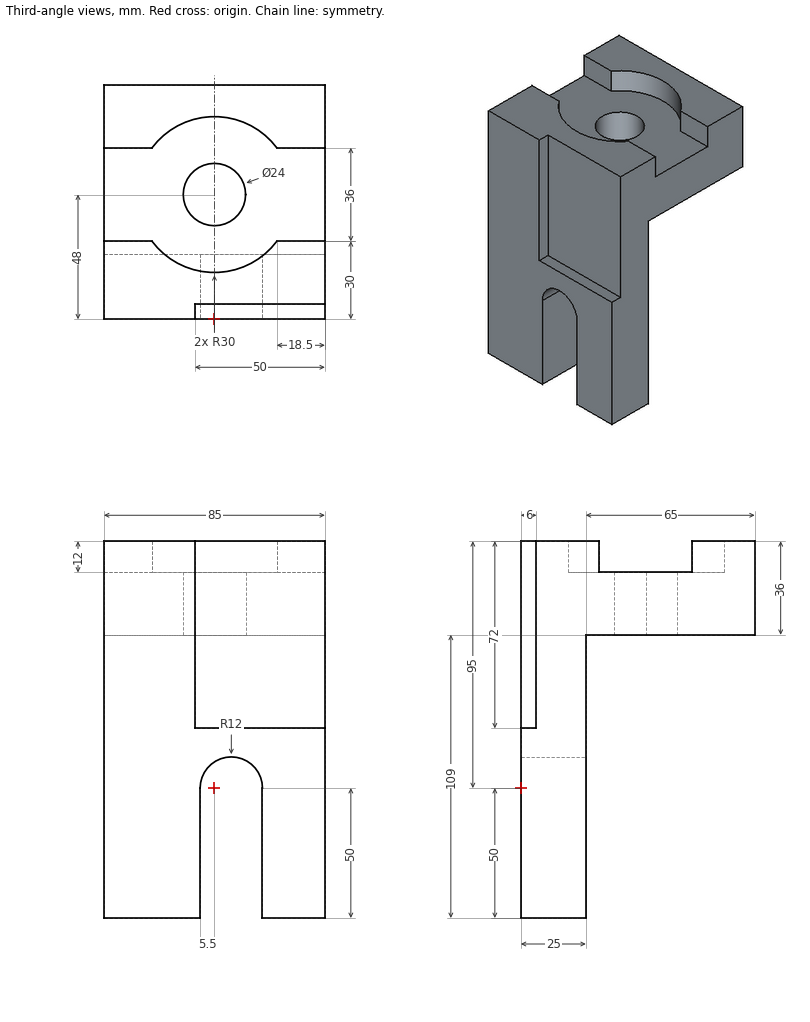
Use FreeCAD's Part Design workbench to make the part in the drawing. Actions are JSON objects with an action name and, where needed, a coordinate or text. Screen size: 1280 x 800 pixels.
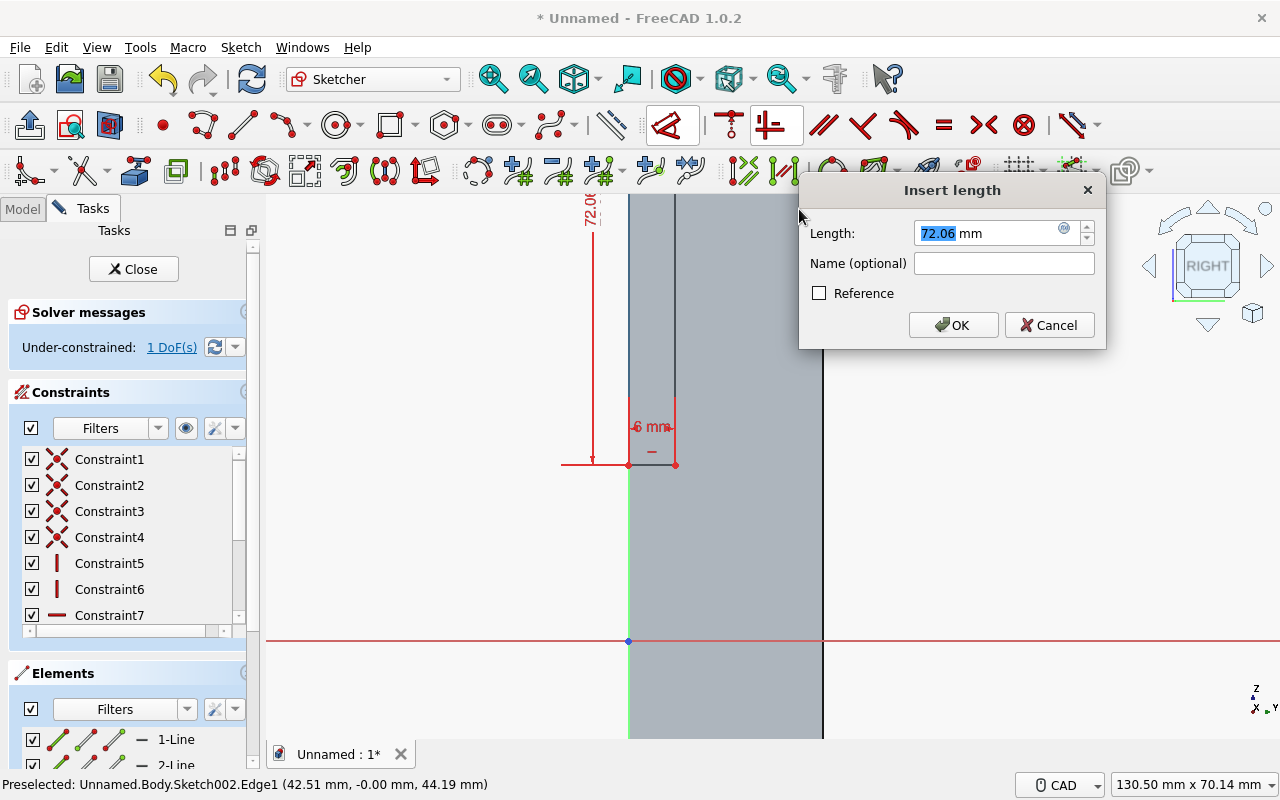
{"action": "type", "text": "72"}
{"action": "key", "text": "Return"}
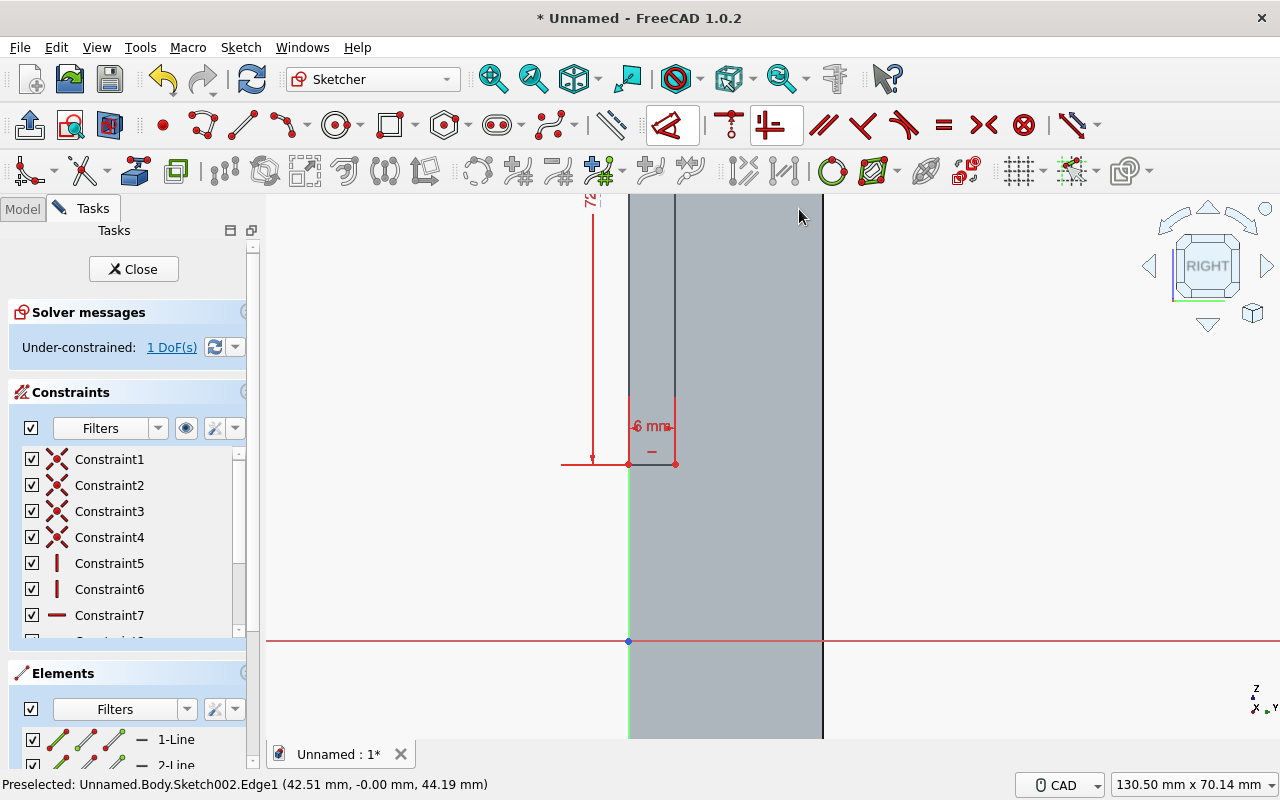
{"action": "scroll", "coordinate": [747, 625], "scroll_direction": "down", "scroll_amount": 4}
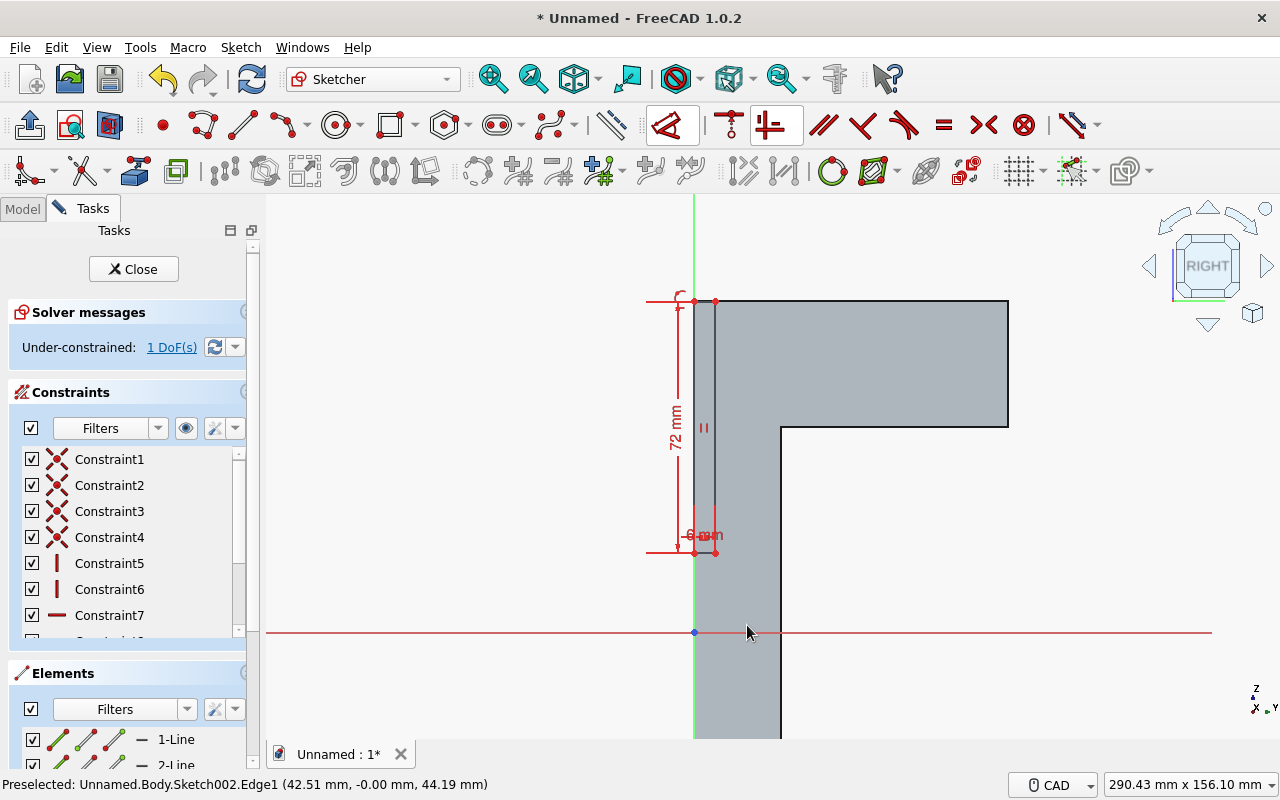
{"action": "left_click", "coordinate": [694, 302]}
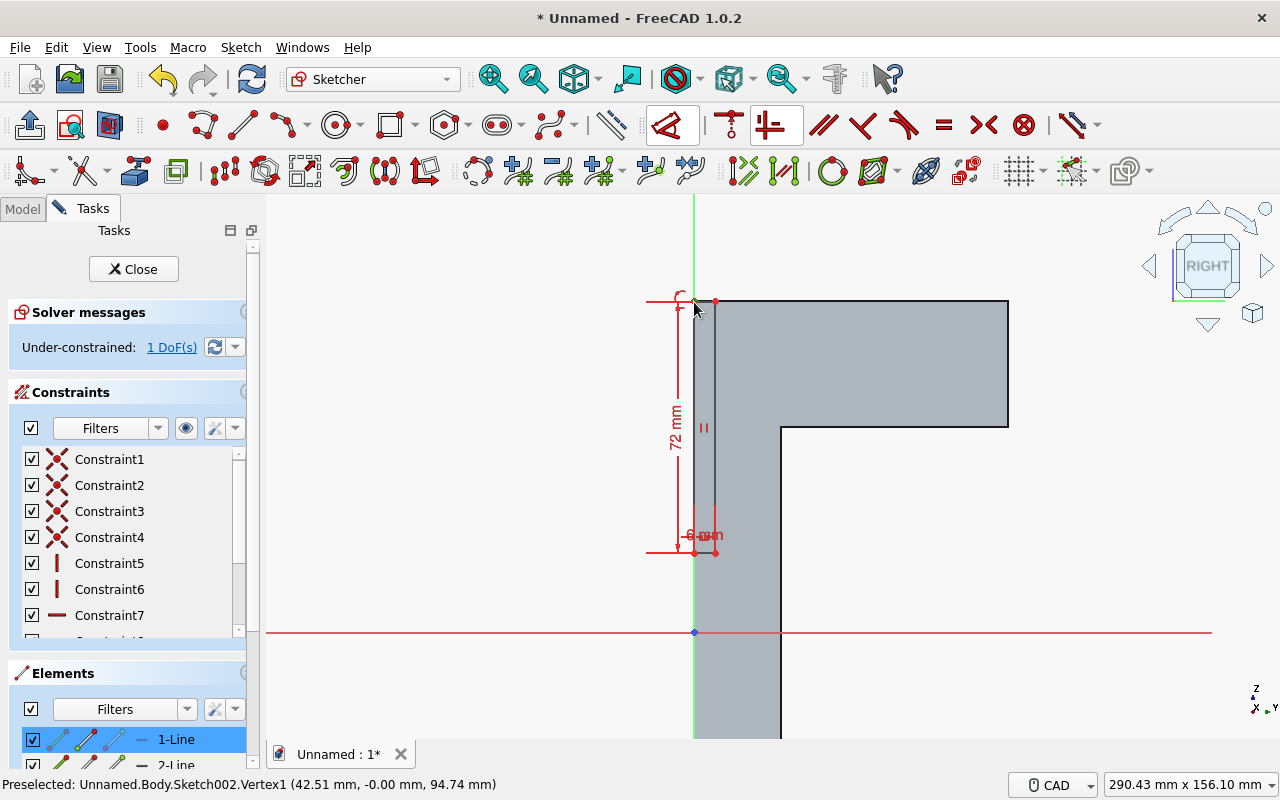
{"action": "left_click", "coordinate": [694, 126]}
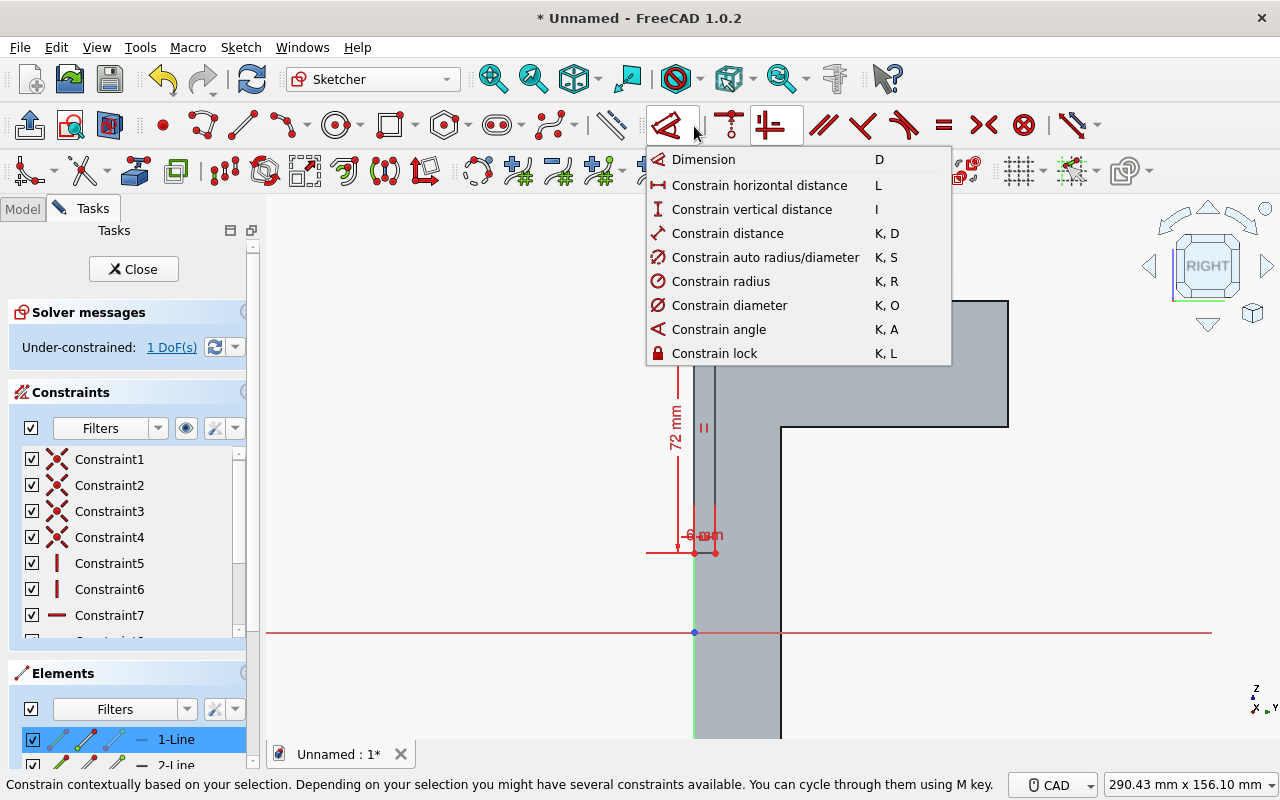
{"action": "left_click", "coordinate": [799, 209]}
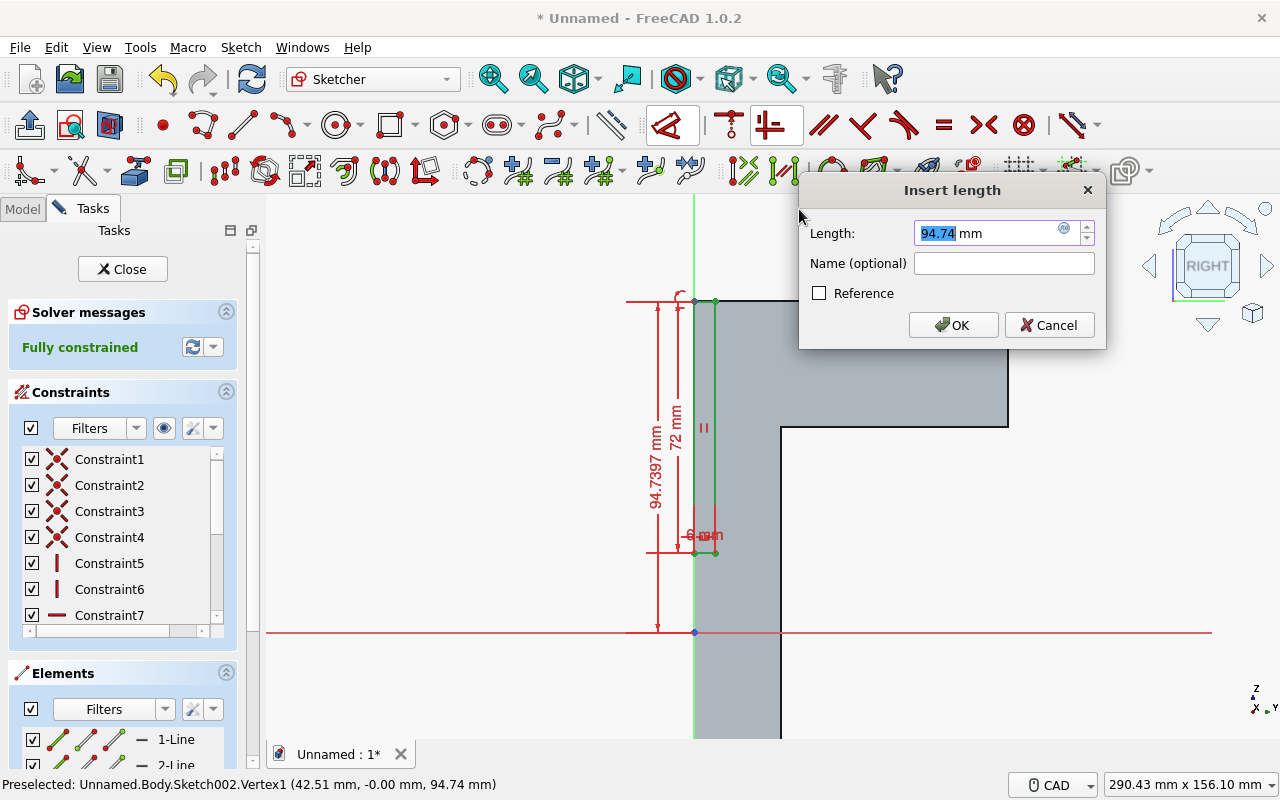
{"action": "type", "text": "95"}
{"action": "key", "text": "Return"}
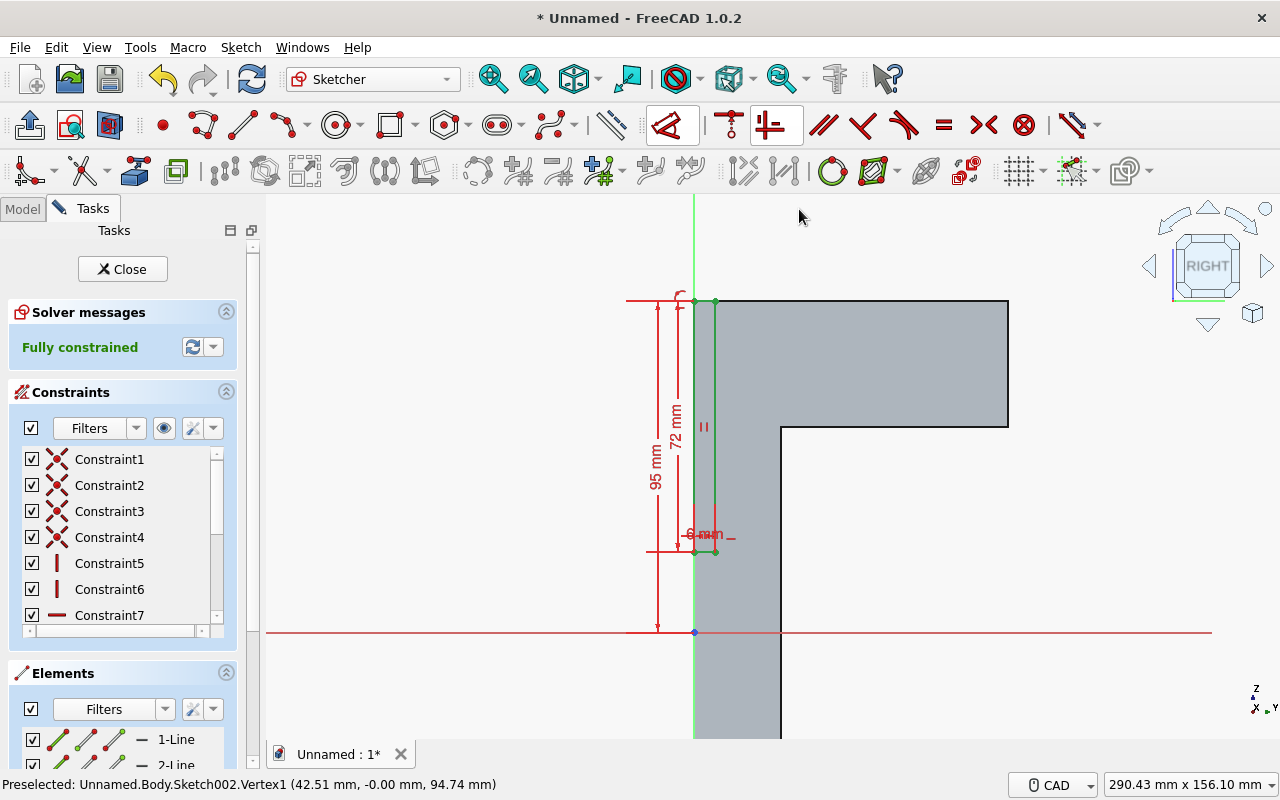
{"action": "left_click", "coordinate": [123, 269]}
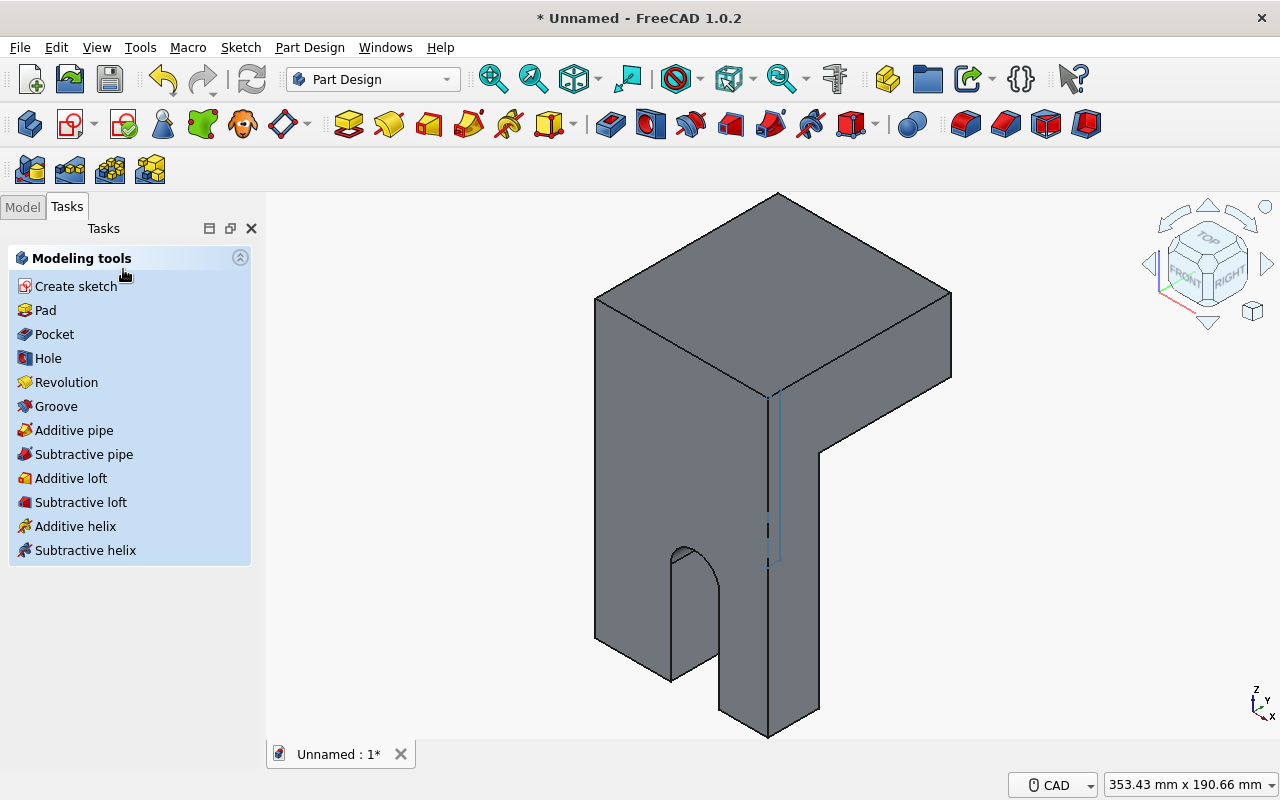
{"action": "left_click", "coordinate": [612, 124]}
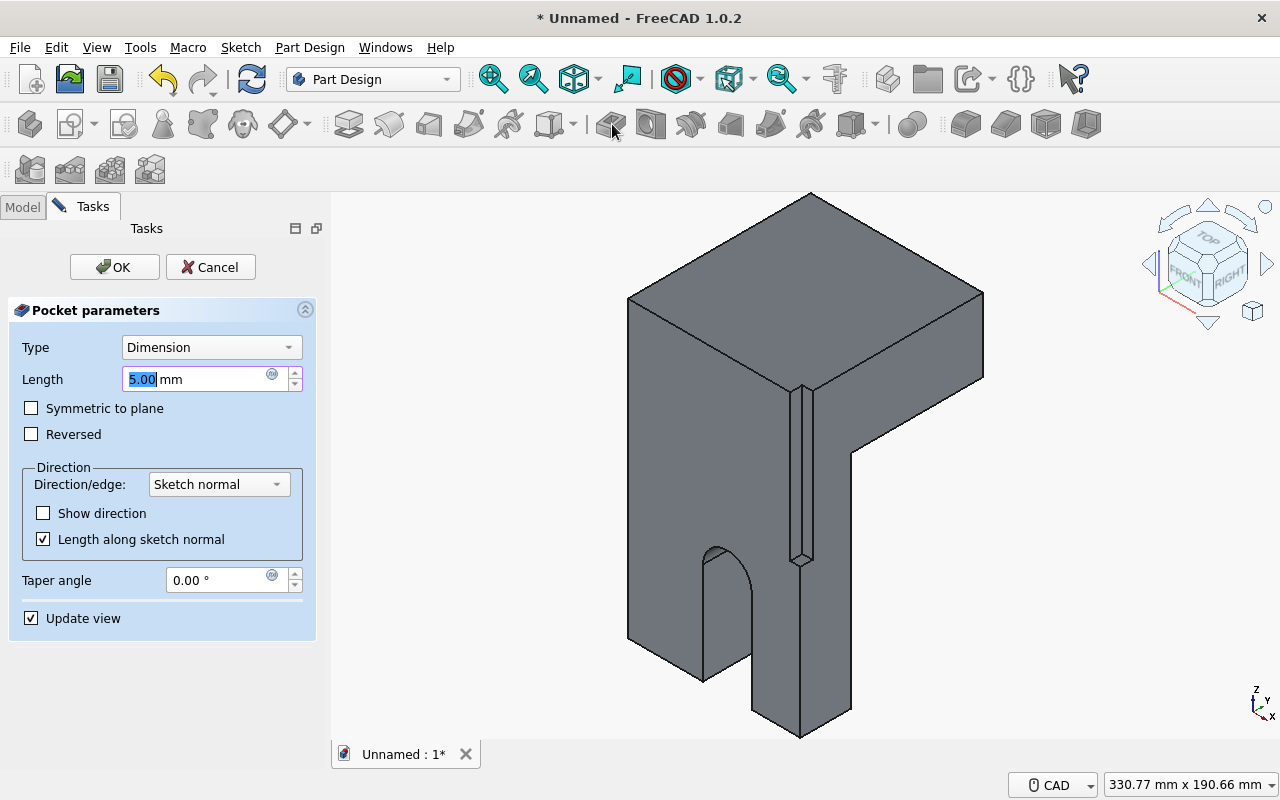
{"action": "type", "text": "50"}
{"action": "key", "text": "Tab"}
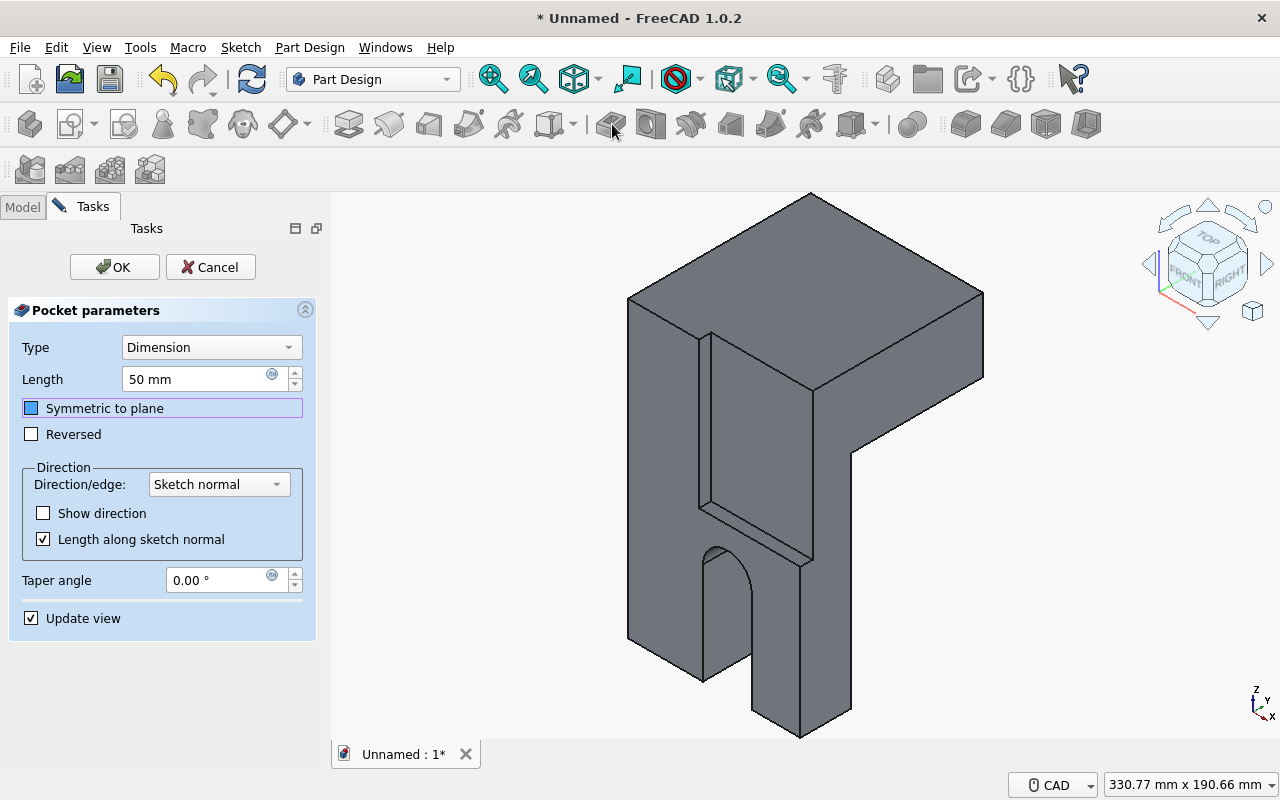
{"action": "left_click", "coordinate": [115, 267]}